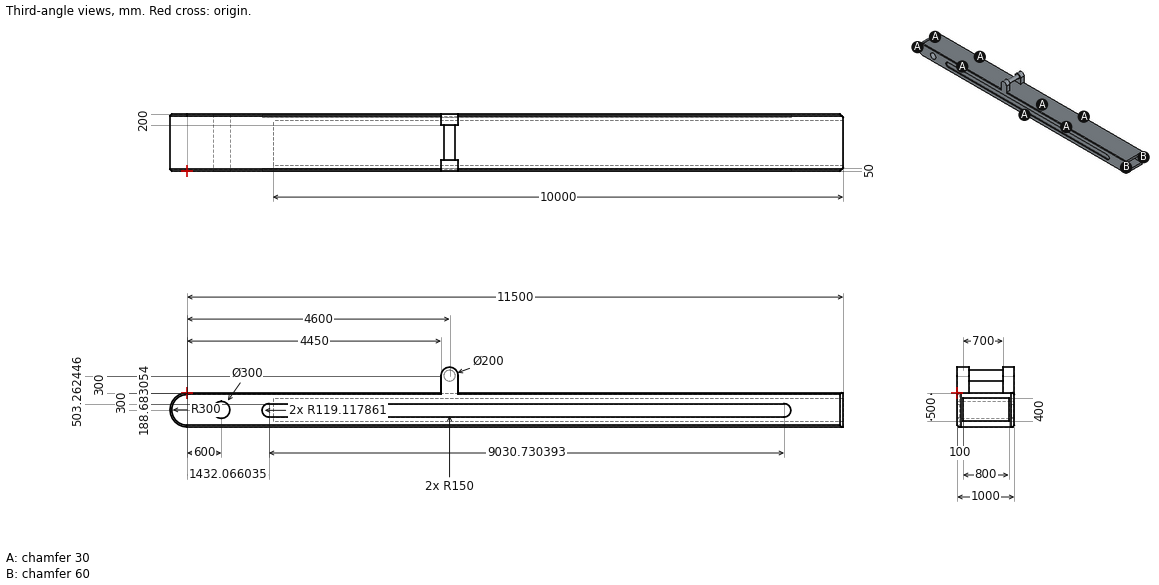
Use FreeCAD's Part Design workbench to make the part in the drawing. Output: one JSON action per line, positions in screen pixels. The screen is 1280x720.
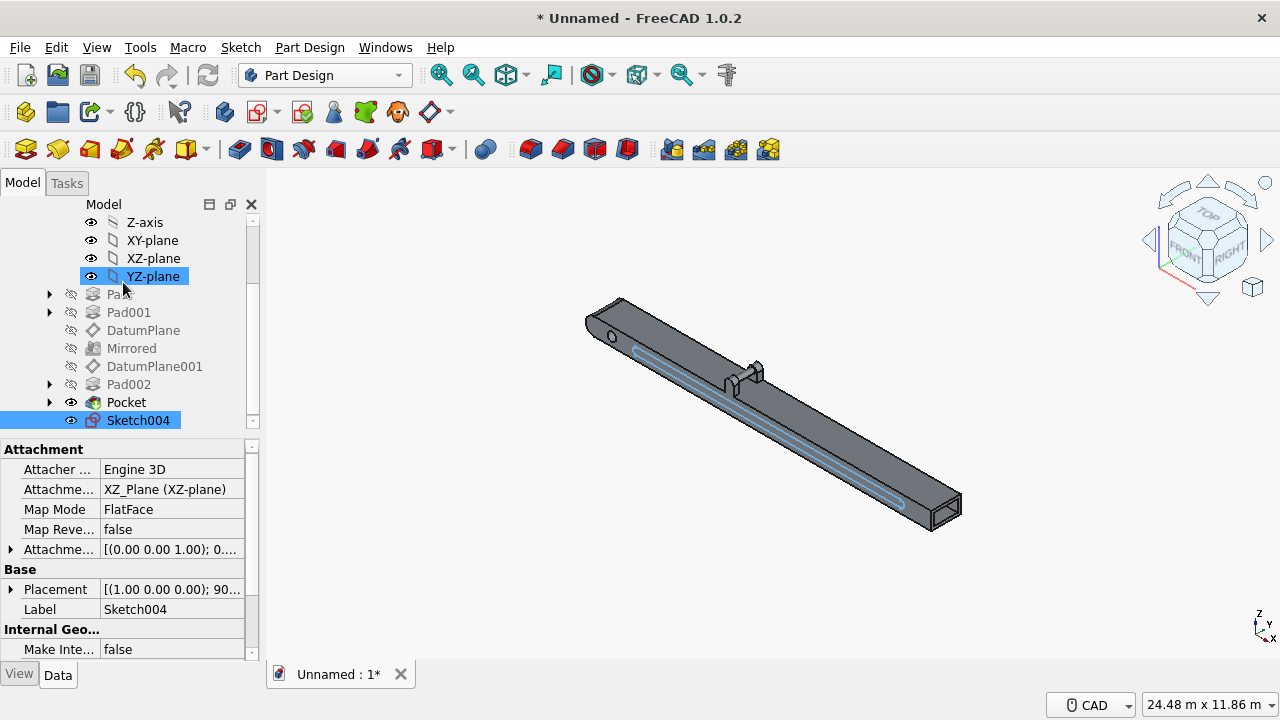
{"action": "left_click", "coordinate": [240, 150]}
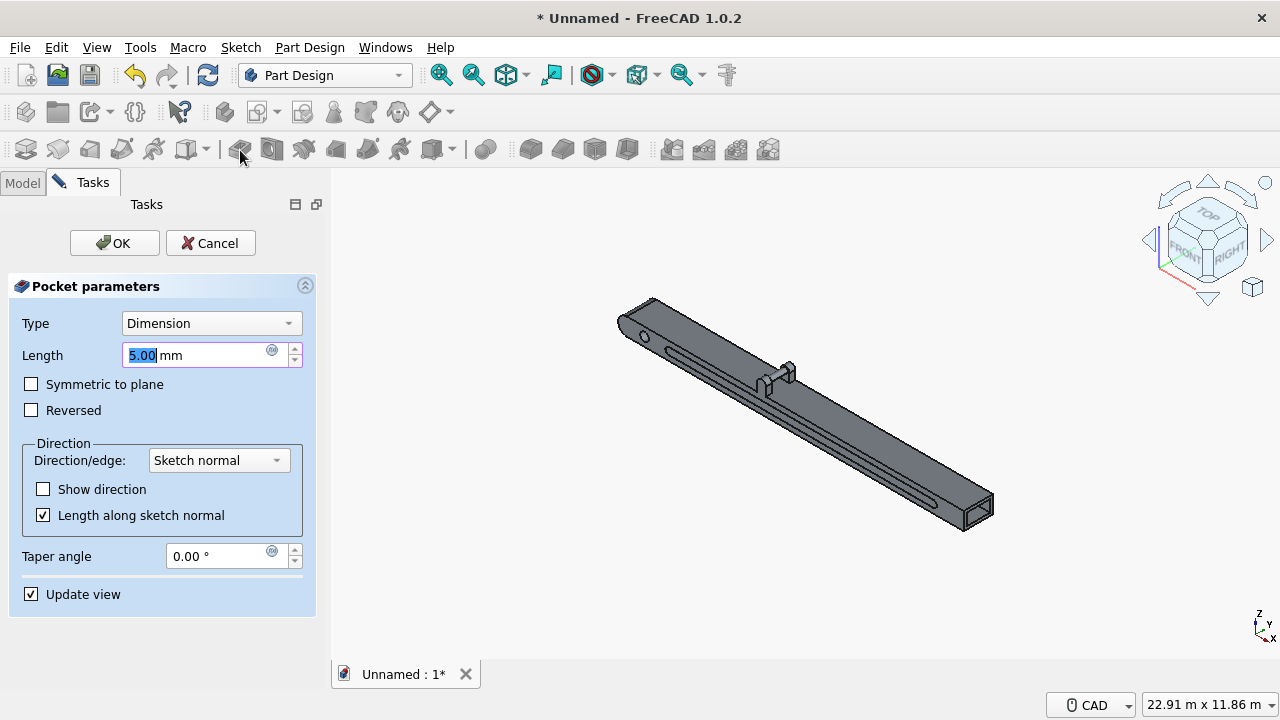
{"action": "type", "text": "50"}
{"action": "key", "text": "Tab"}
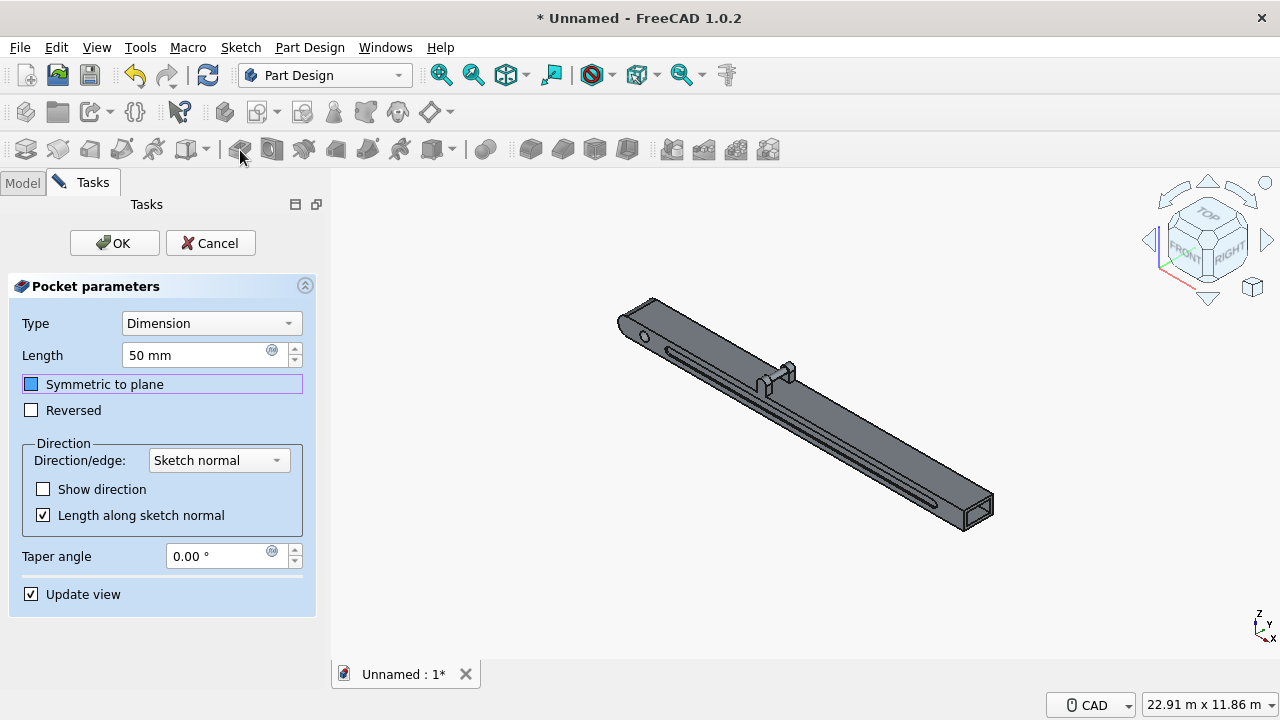
{"action": "left_click", "coordinate": [115, 243]}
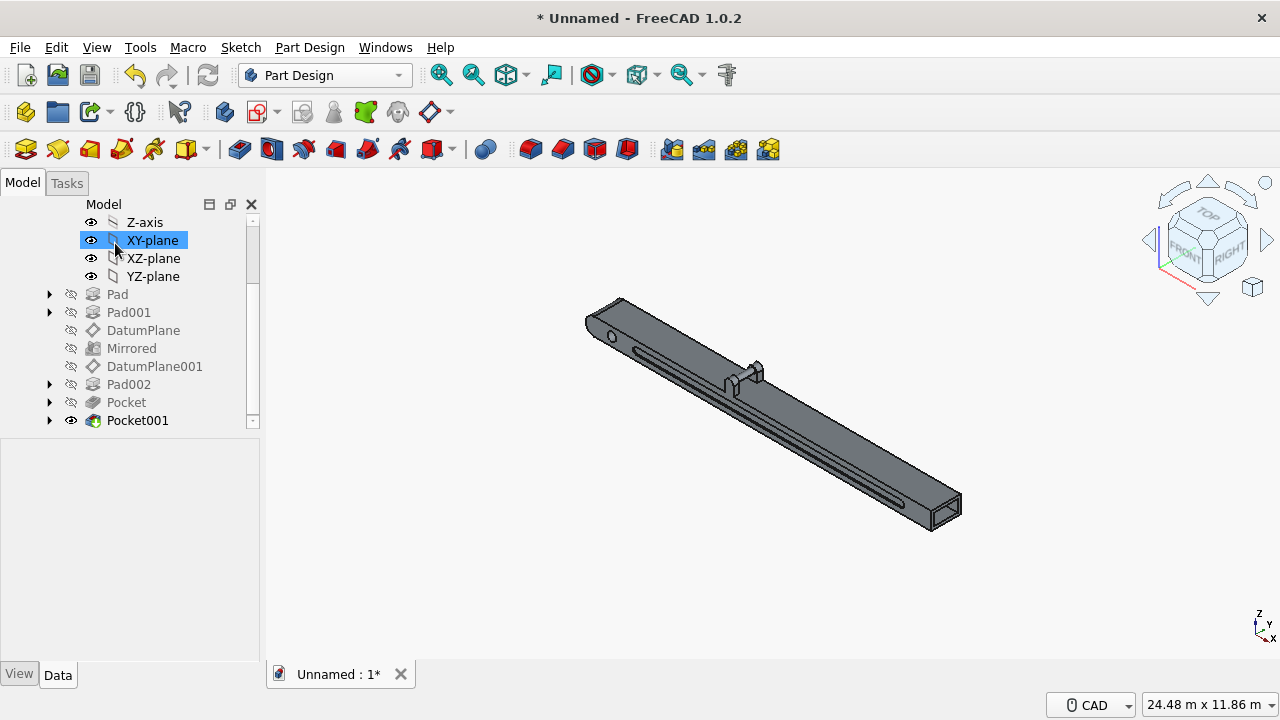
{"action": "scroll", "coordinate": [160, 326], "scroll_direction": "down", "scroll_amount": 3}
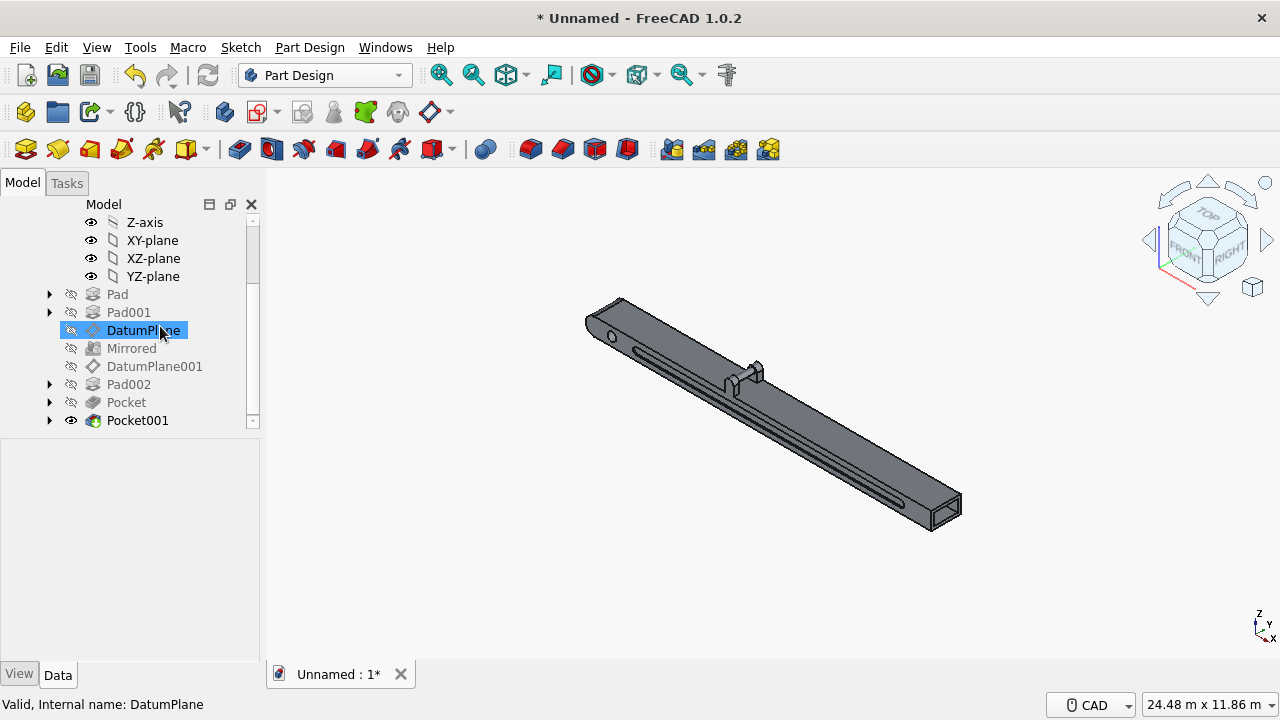
{"action": "scroll", "coordinate": [160, 326], "scroll_direction": "up", "scroll_amount": 15}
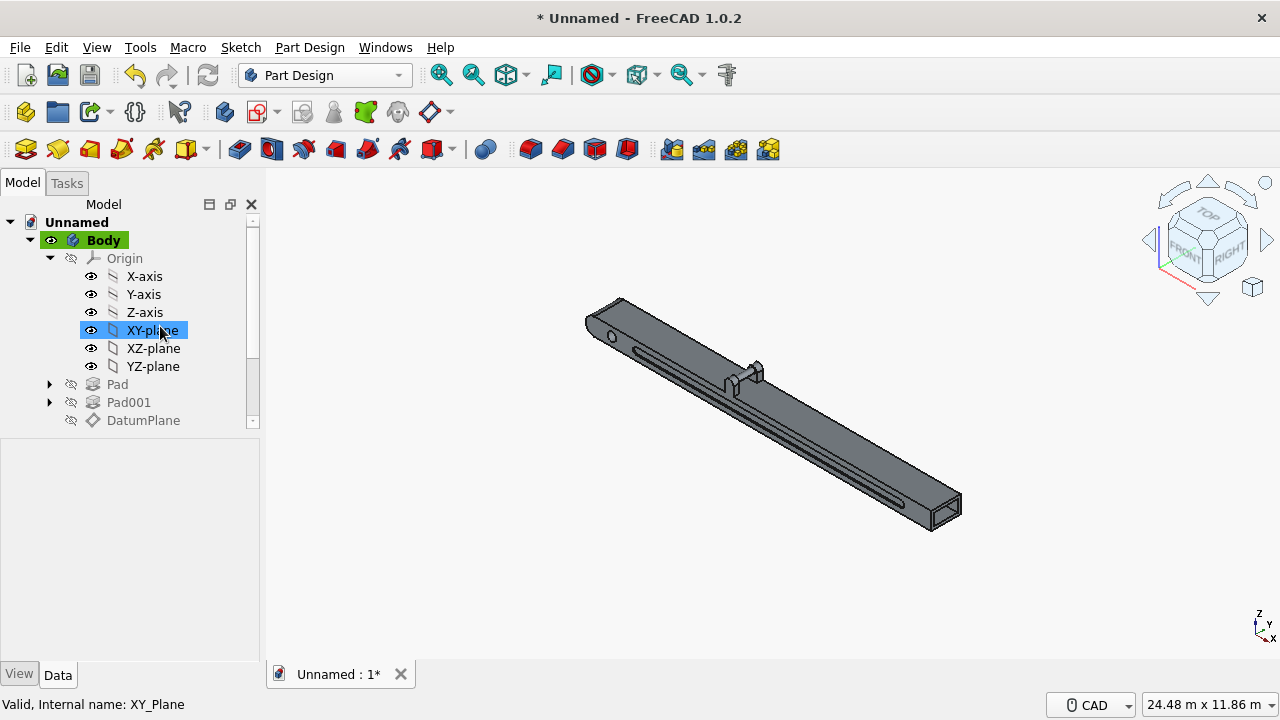
{"action": "left_click", "coordinate": [136, 348]}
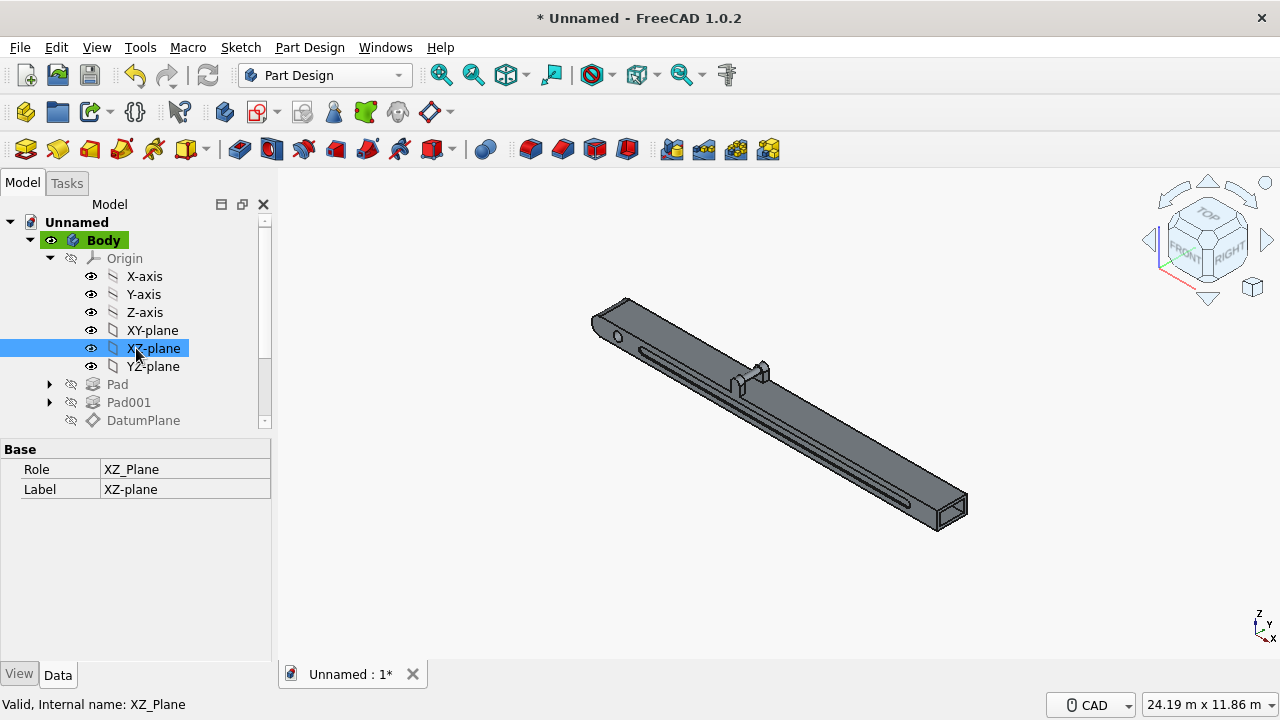
{"action": "left_click", "coordinate": [430, 112]}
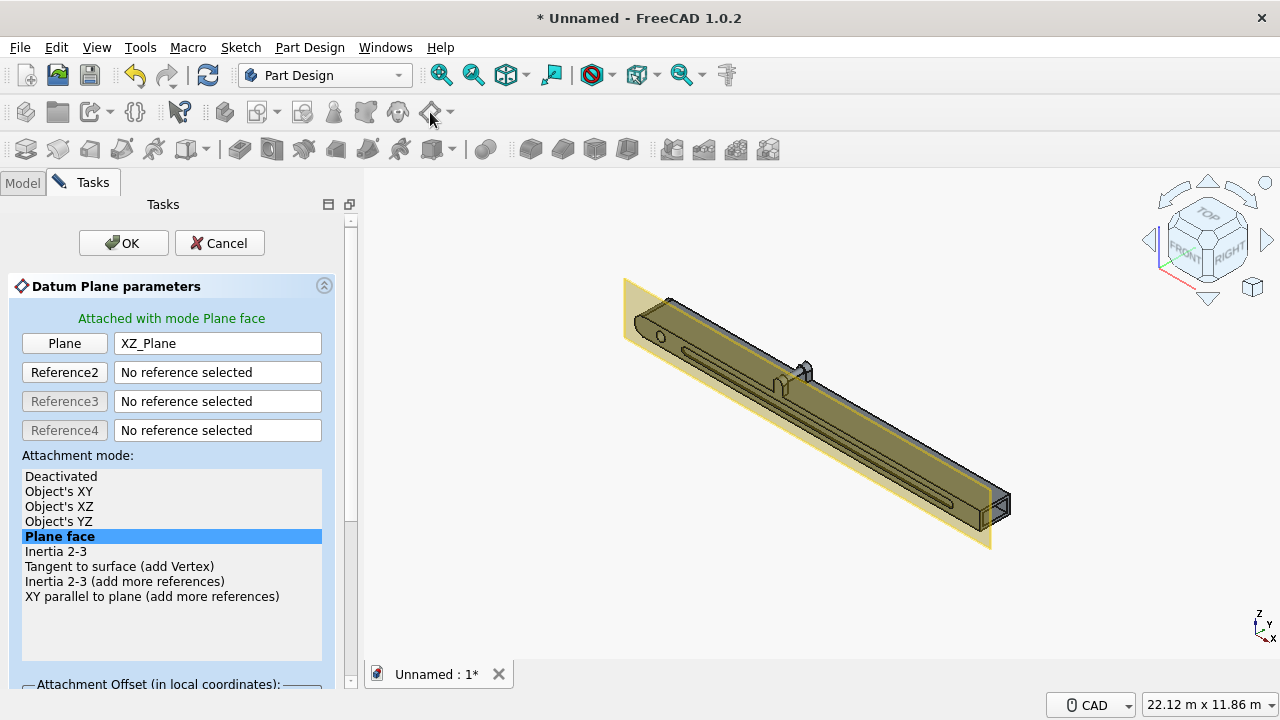
{"action": "scroll", "coordinate": [351, 451], "scroll_direction": "down", "scroll_amount": 3}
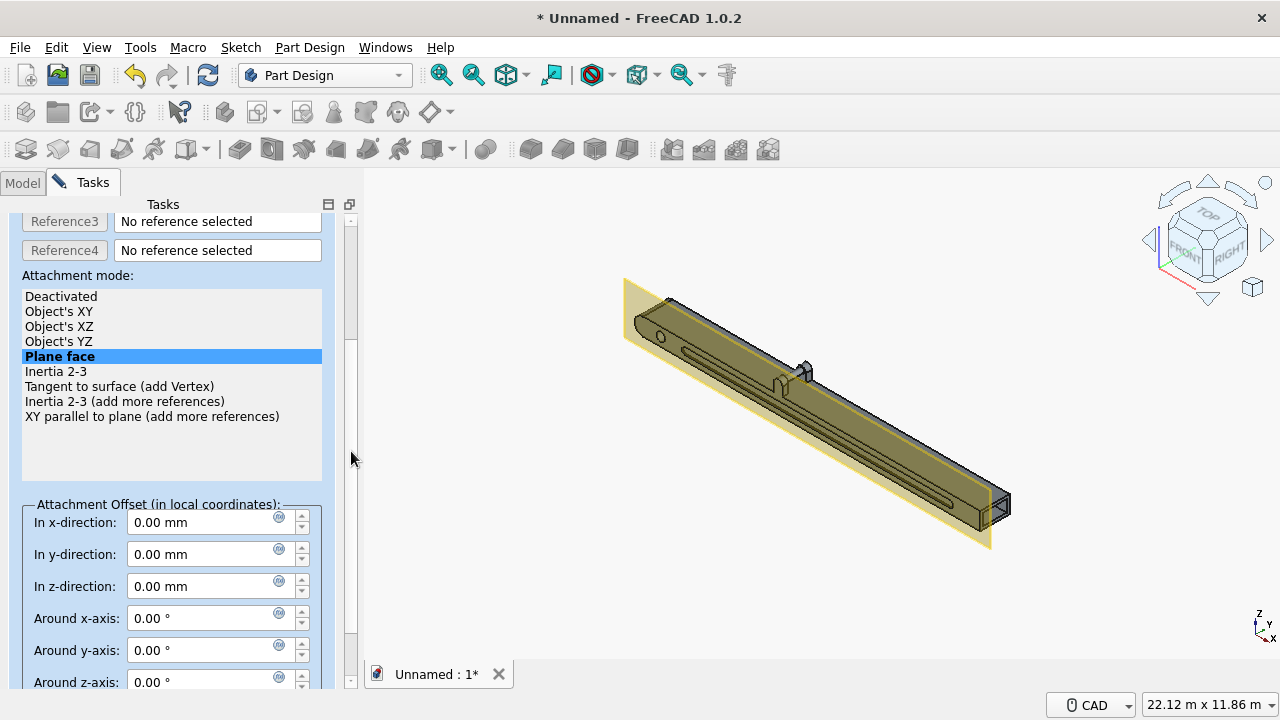
{"action": "triple_click", "coordinate": [210, 586]}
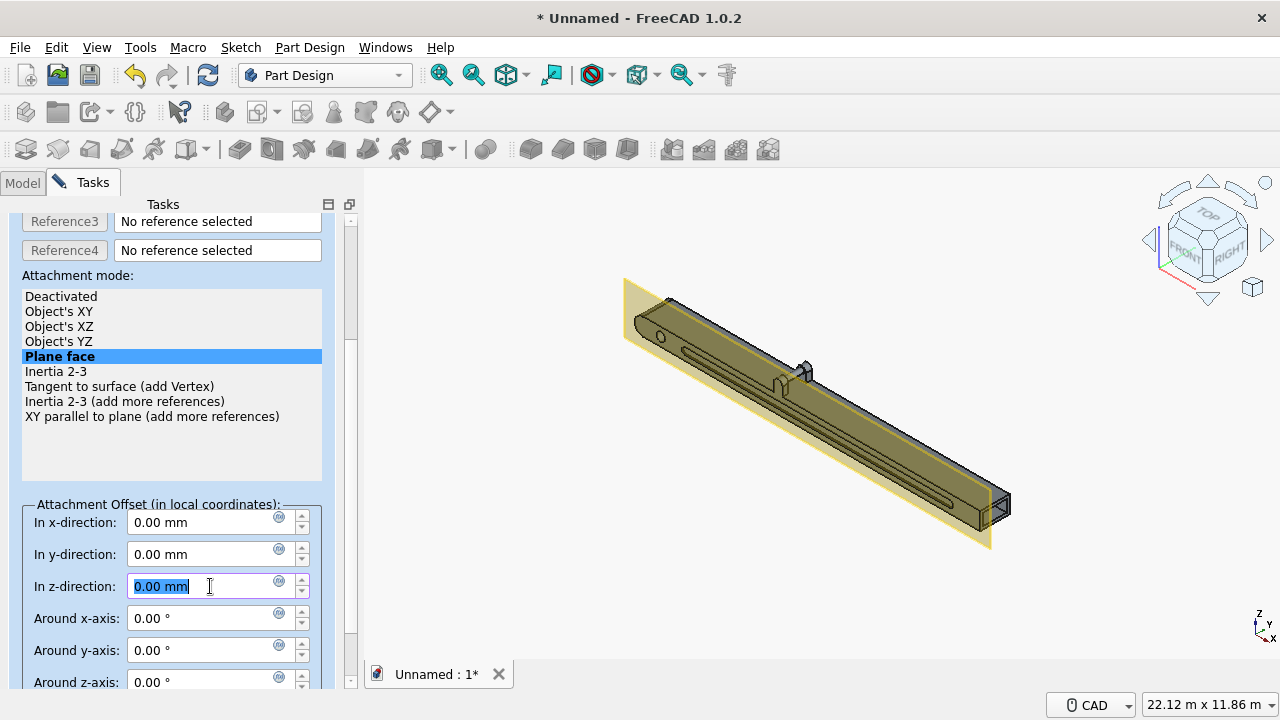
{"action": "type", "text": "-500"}
{"action": "key", "text": "Tab"}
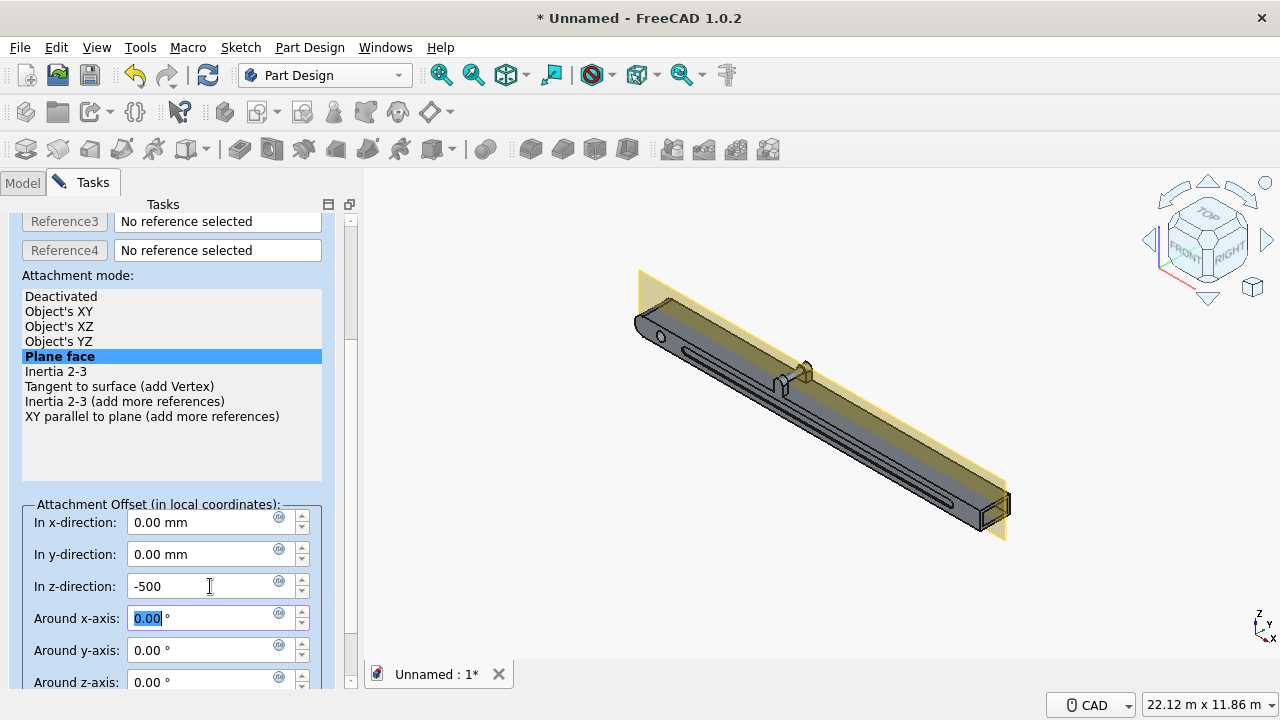
{"action": "scroll", "coordinate": [351, 451], "scroll_direction": "up", "scroll_amount": 4}